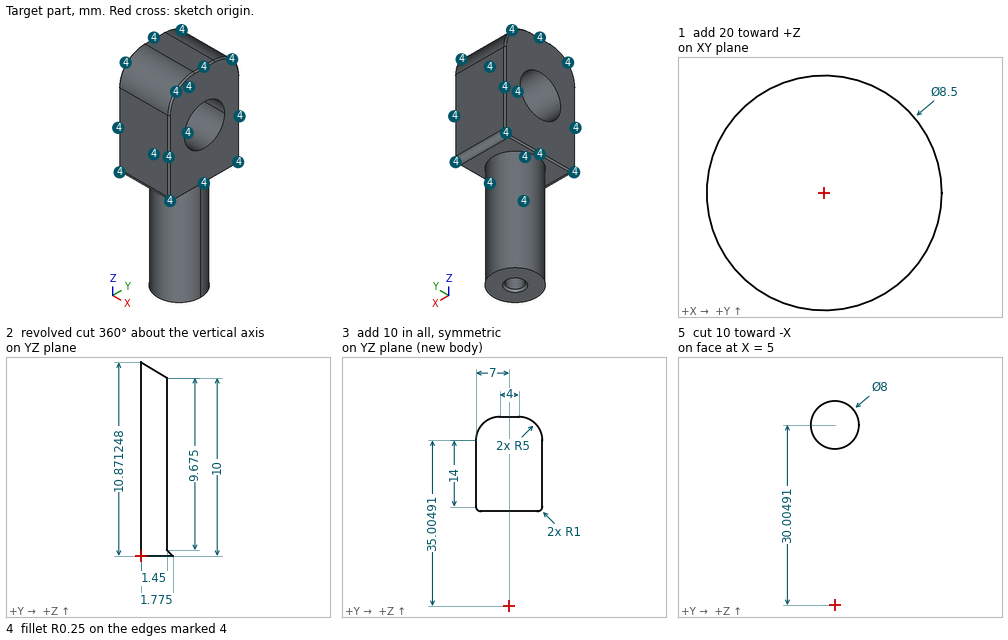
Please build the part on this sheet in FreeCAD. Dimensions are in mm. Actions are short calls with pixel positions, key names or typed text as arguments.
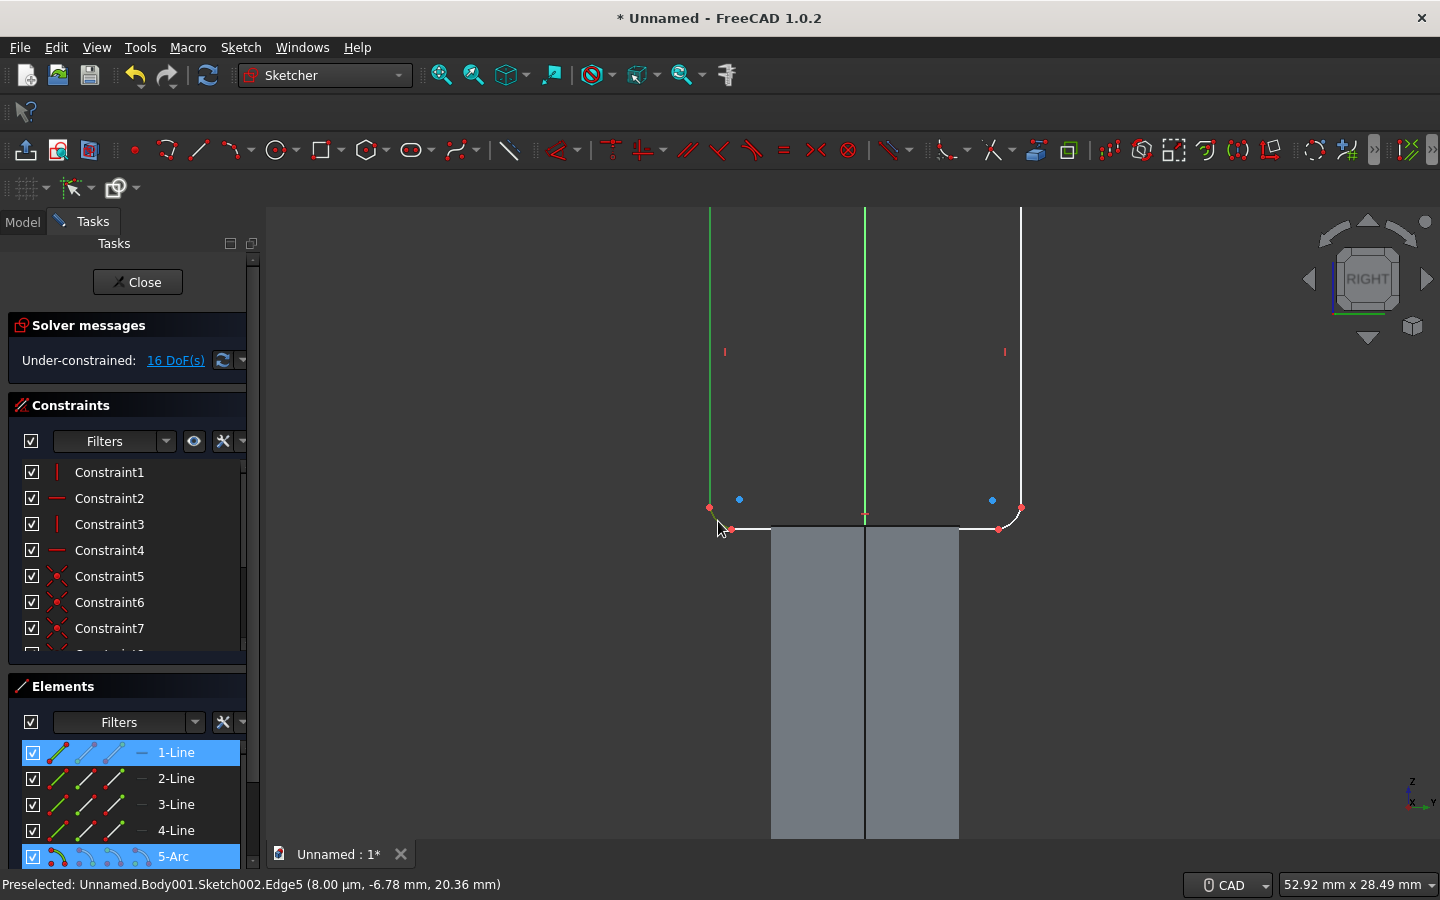
key(t)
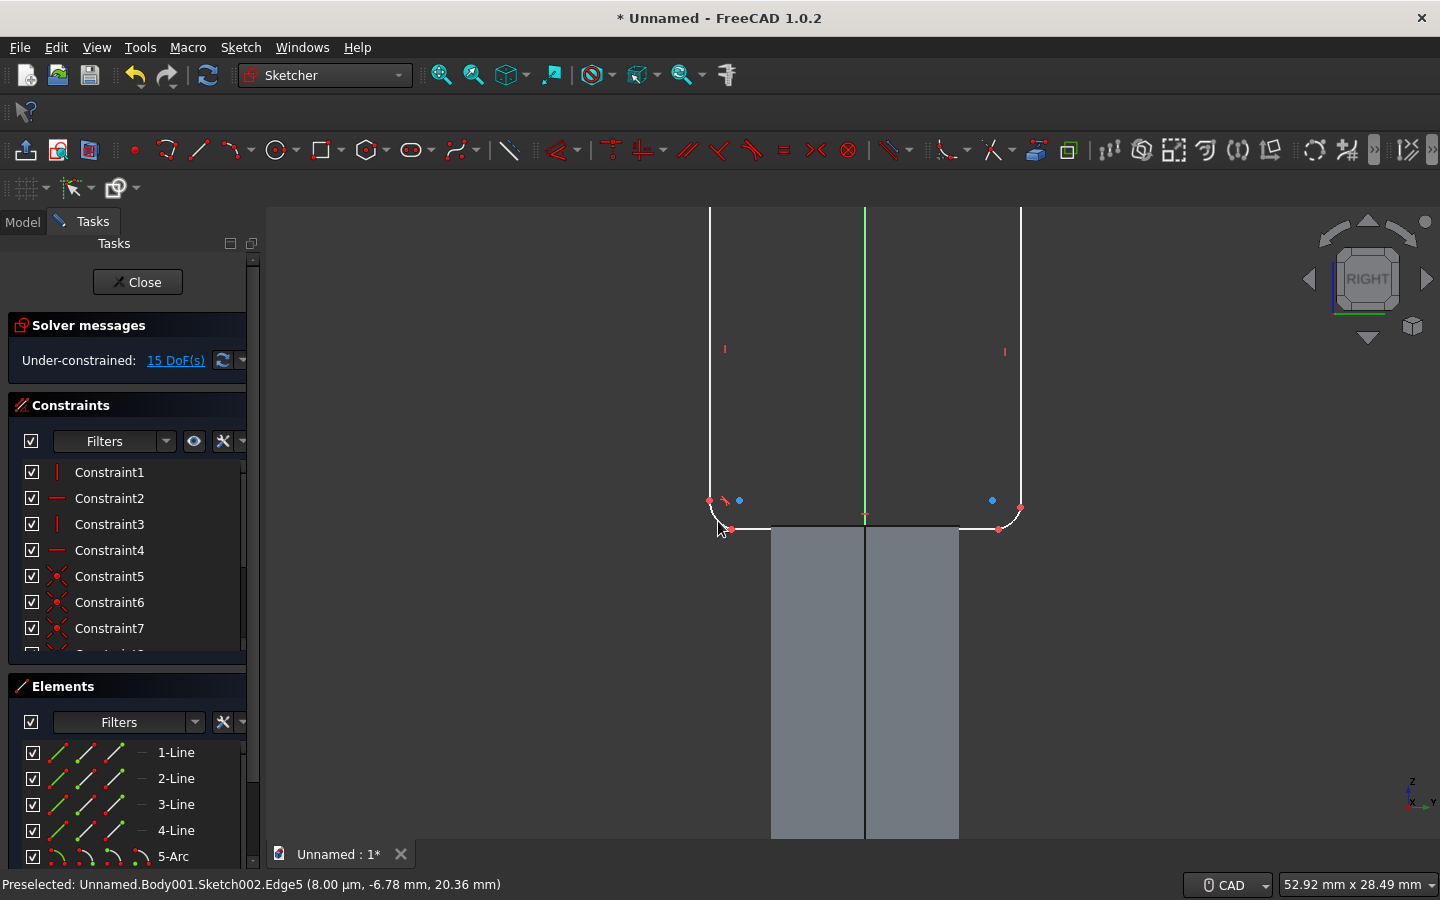
click(710, 287)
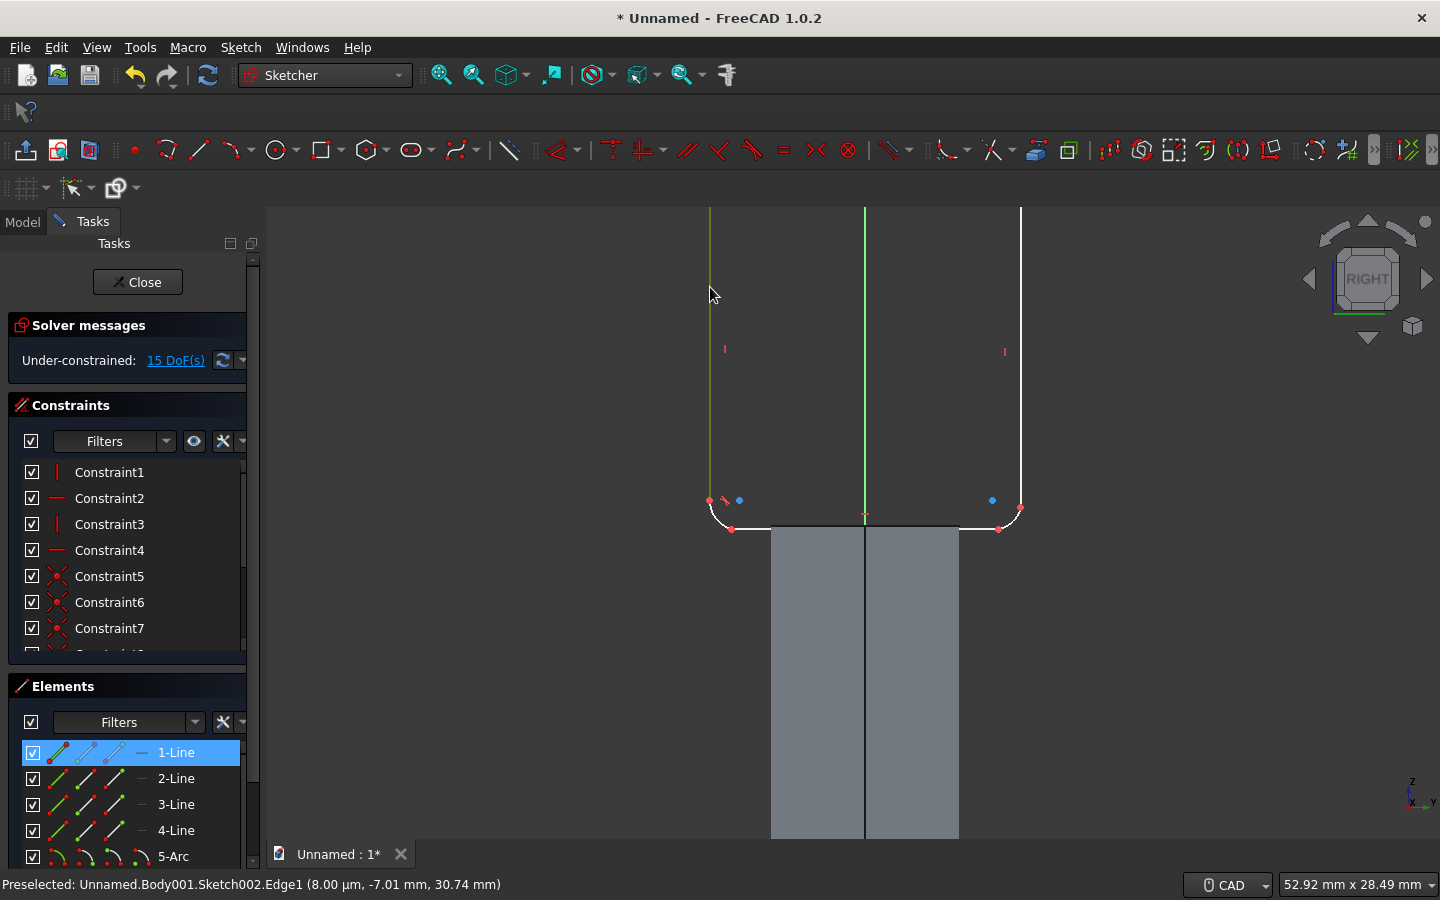
scroll(718, 520, down, 4)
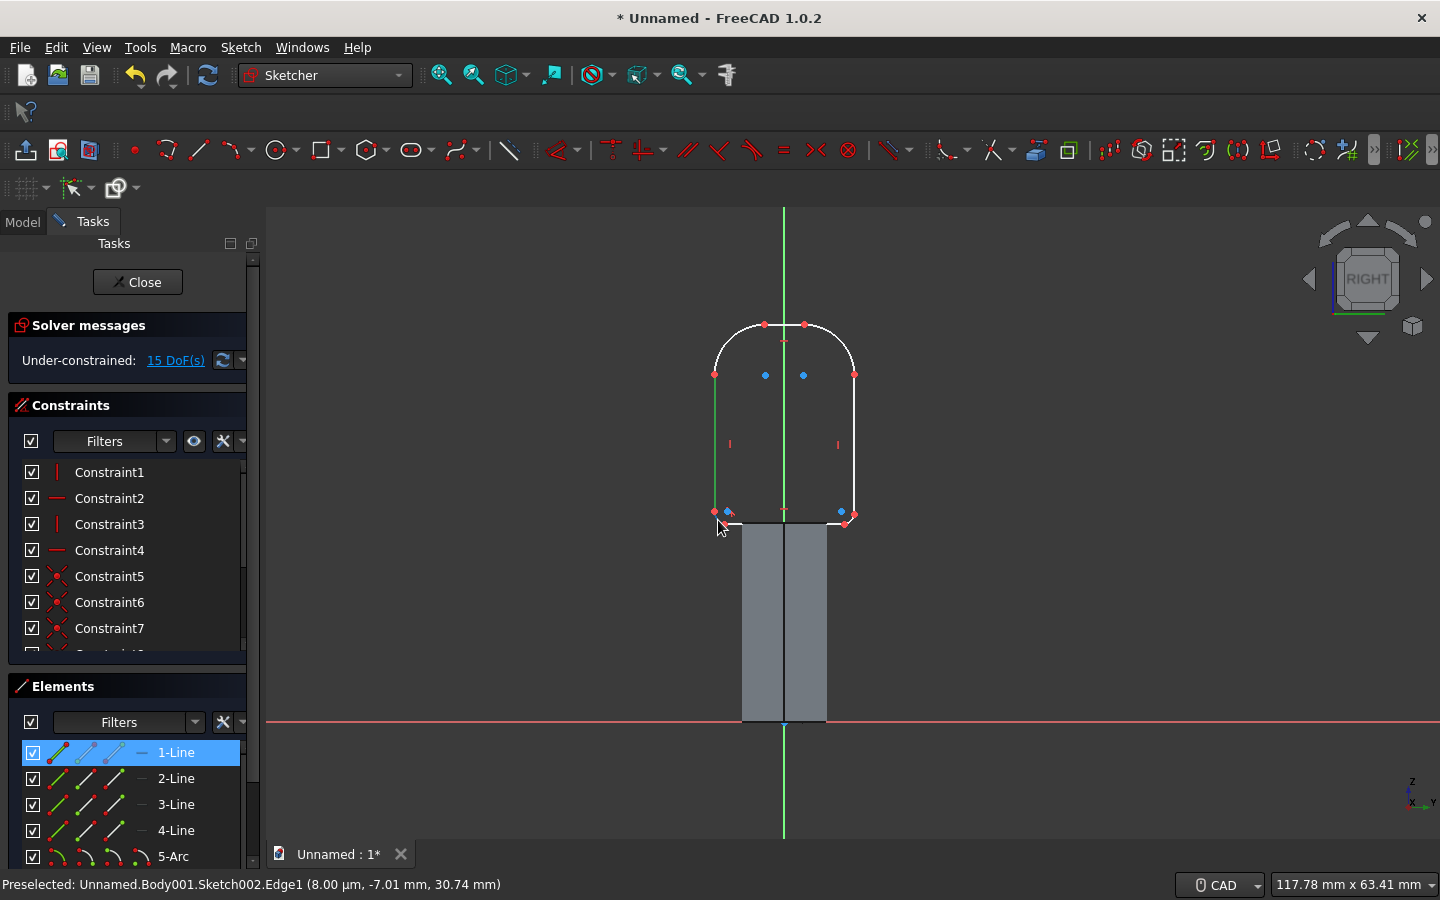
click(742, 330)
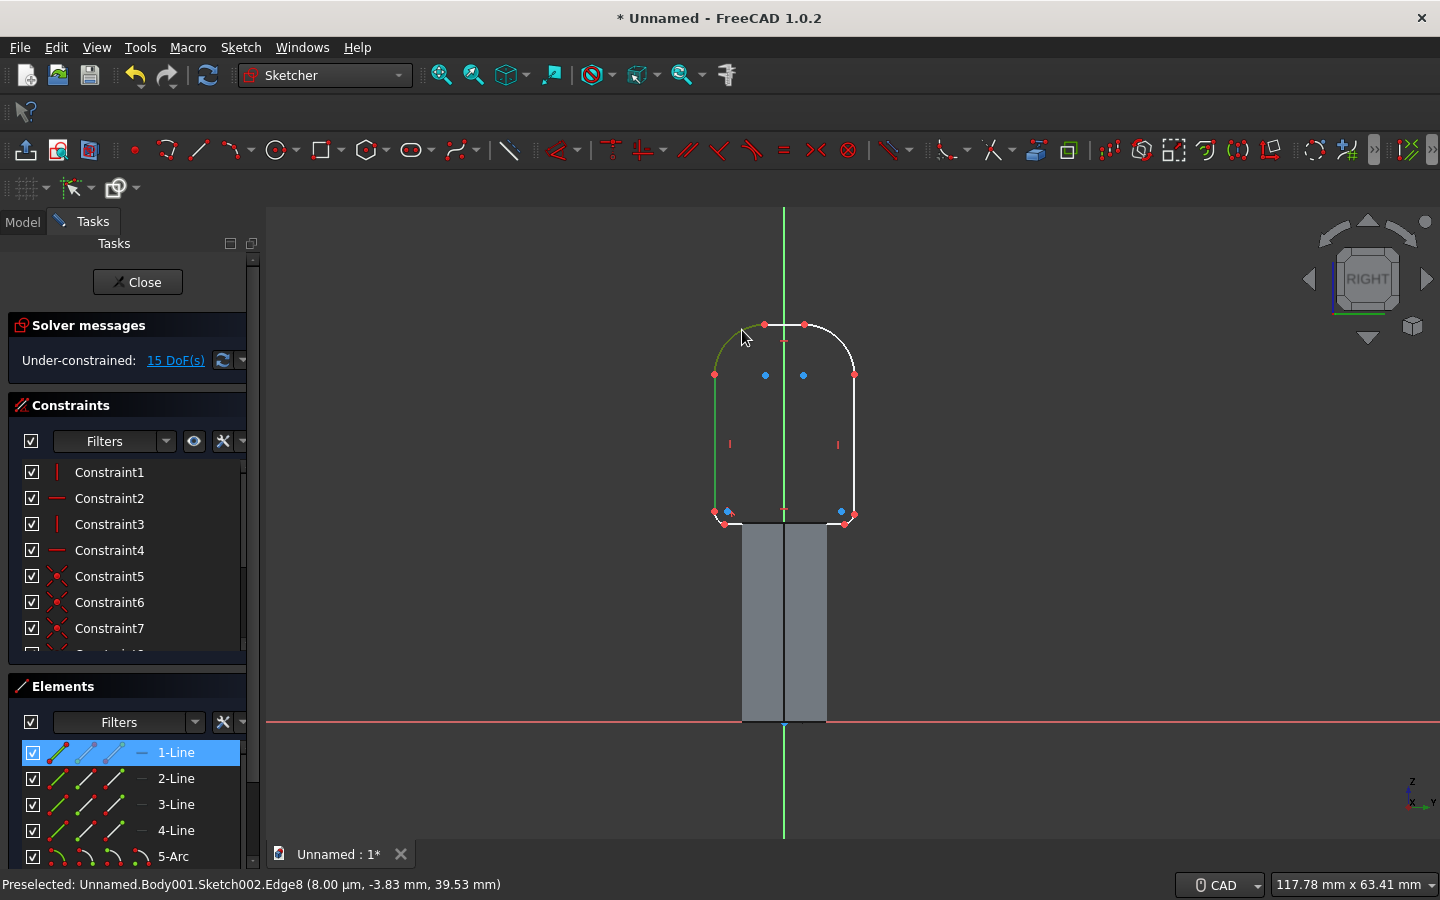
click(752, 150)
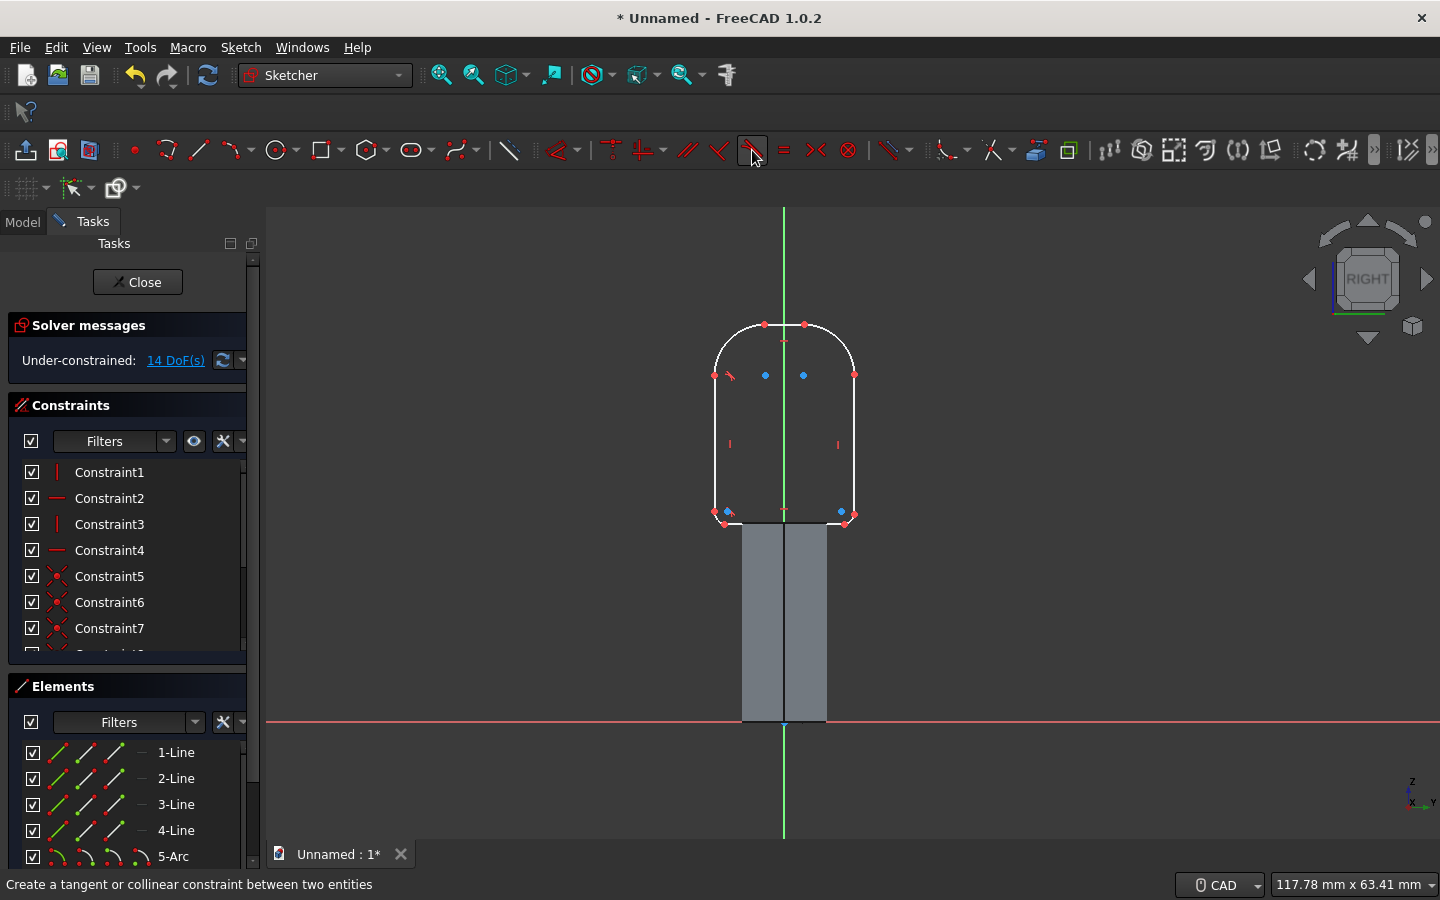
click(760, 524)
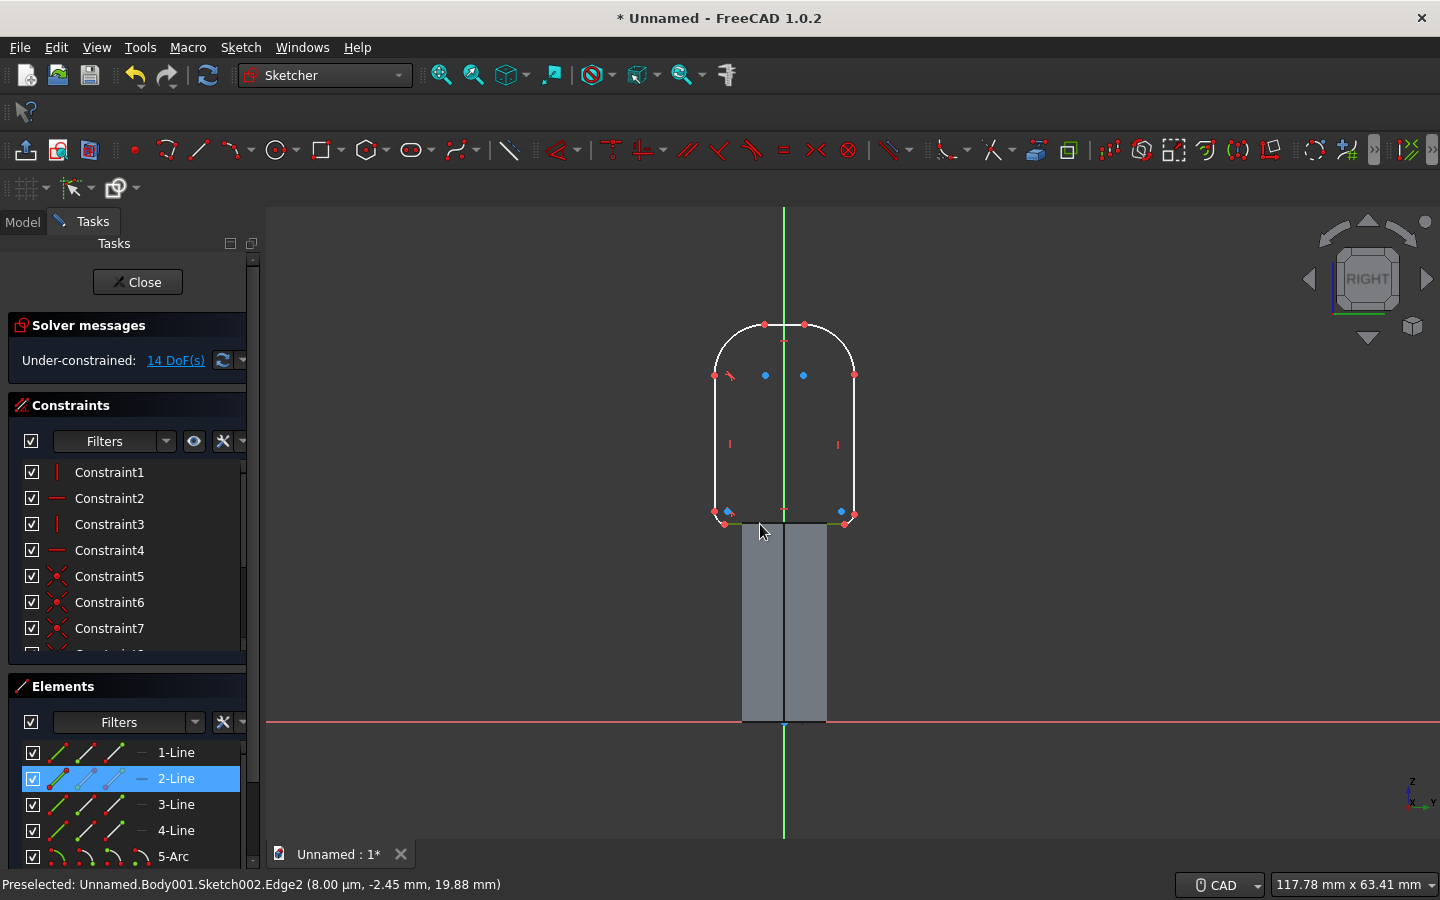
scroll(717, 520, up, 3)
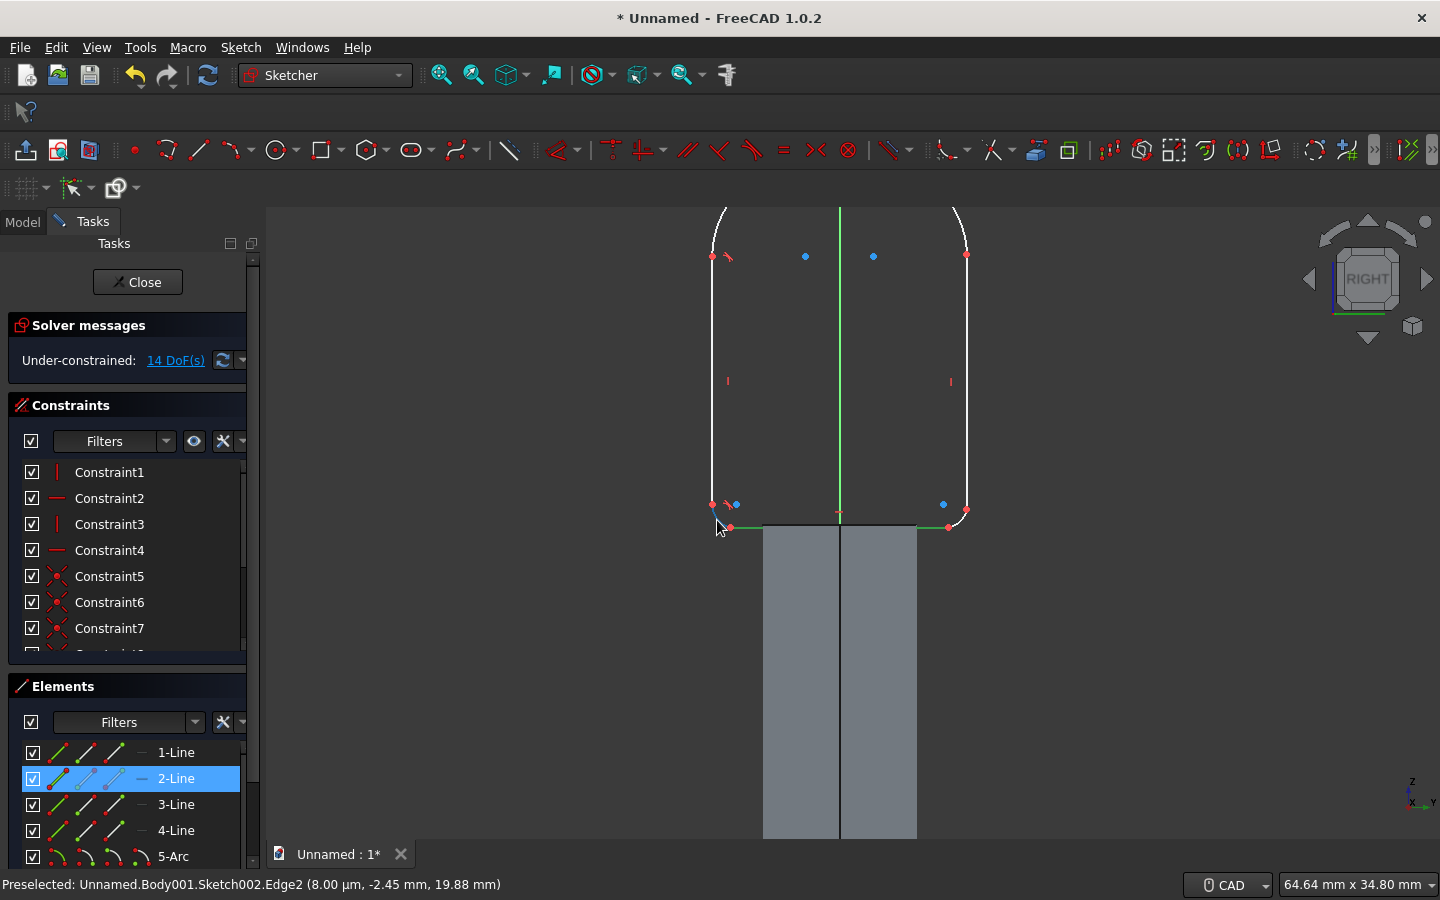
click(717, 519)